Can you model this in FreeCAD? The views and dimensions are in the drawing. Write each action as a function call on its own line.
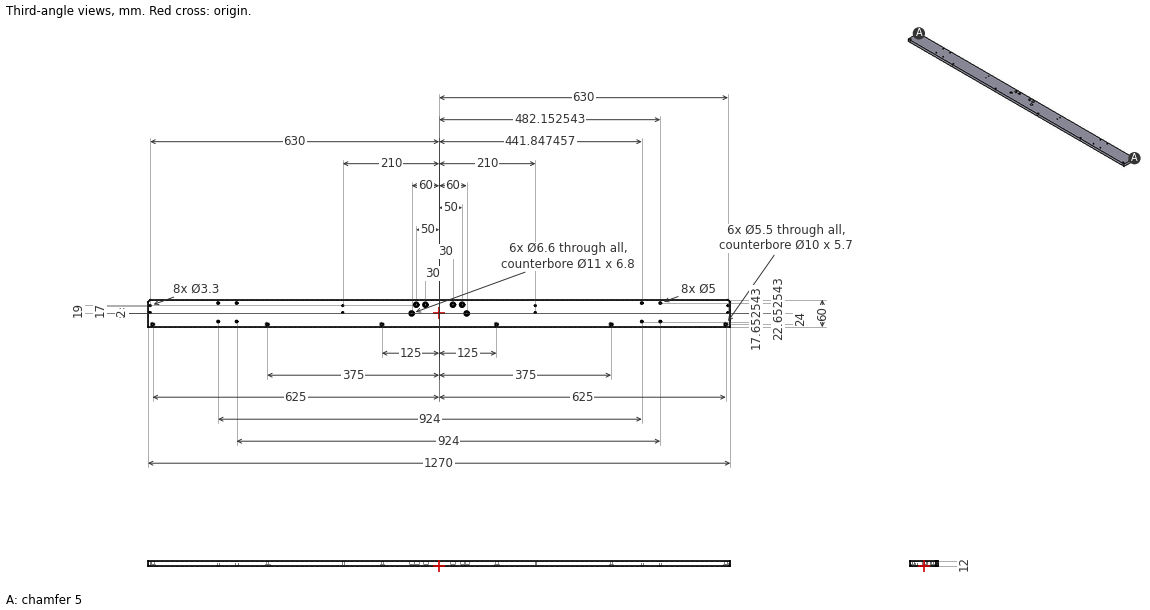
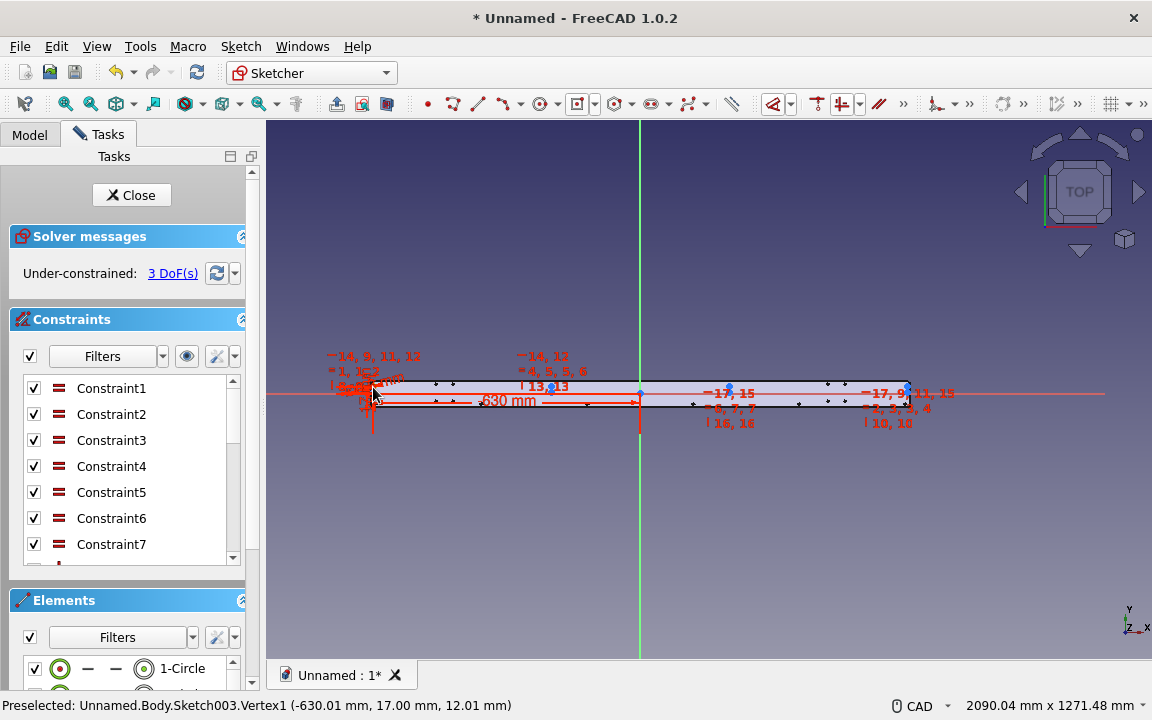
scroll(907, 393, up, 4)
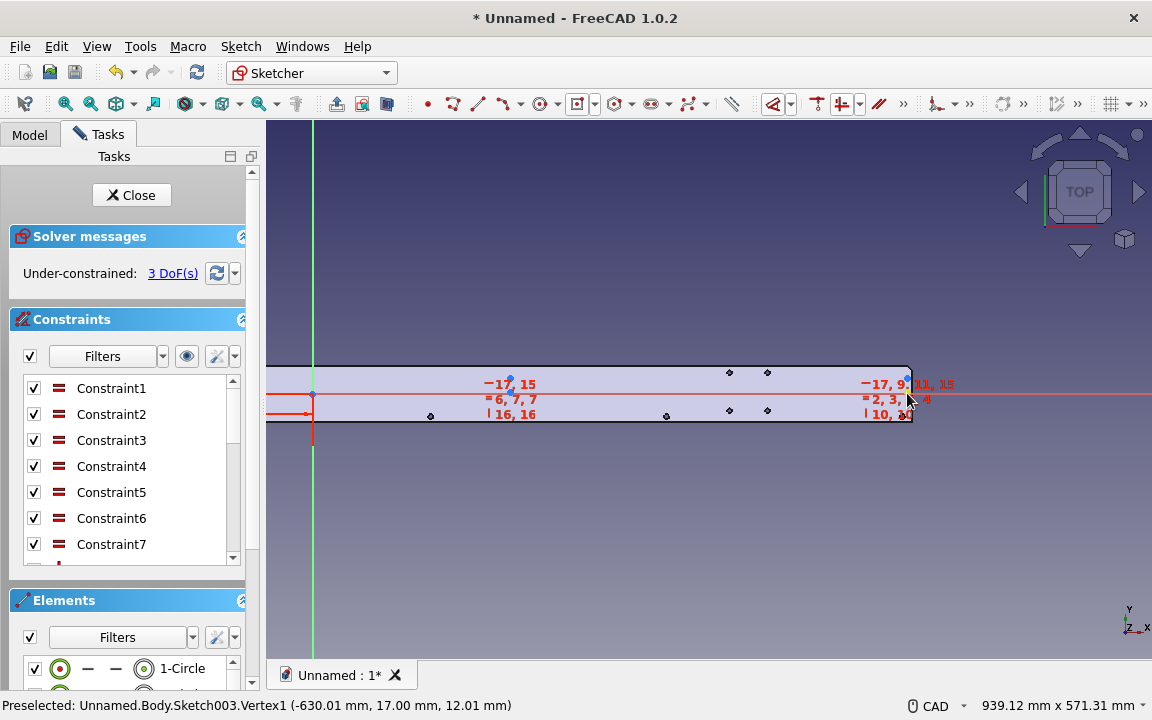
click(907, 392)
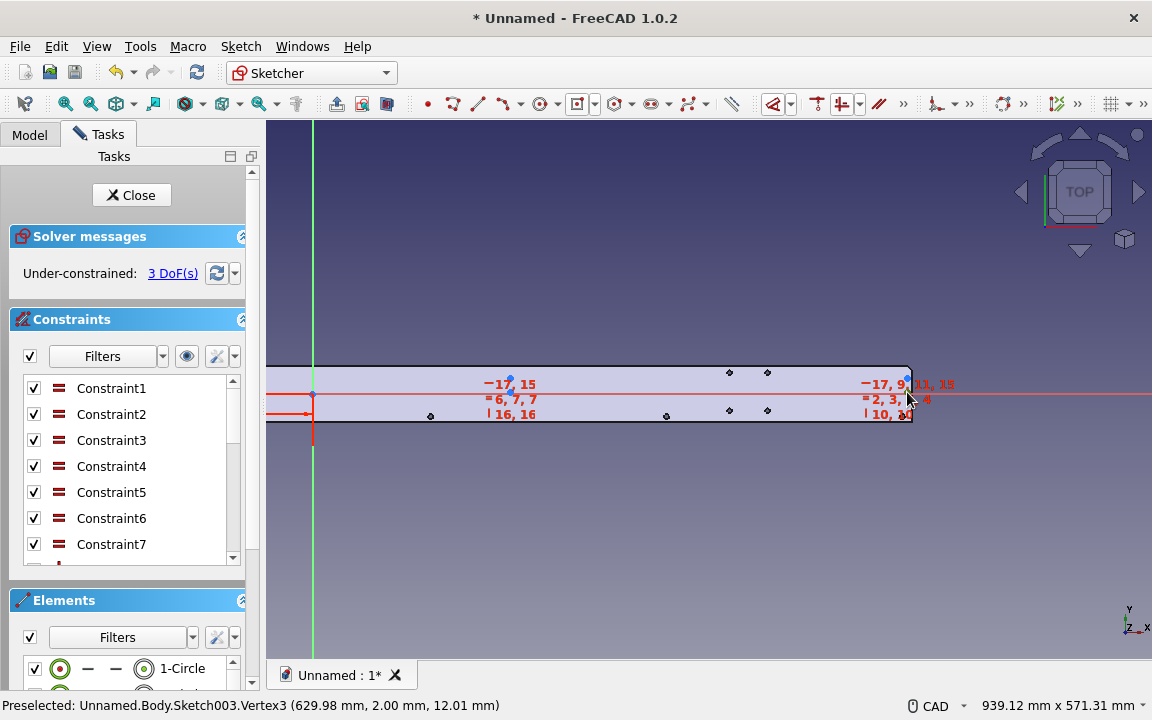
click(790, 104)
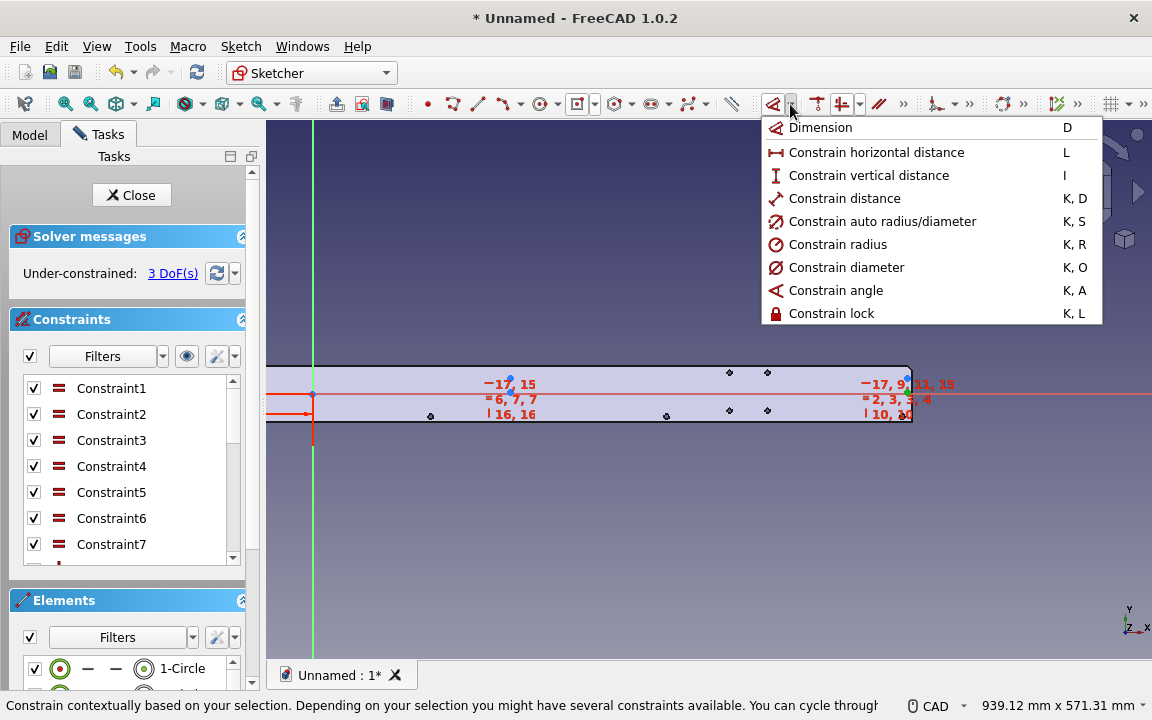
click(932, 152)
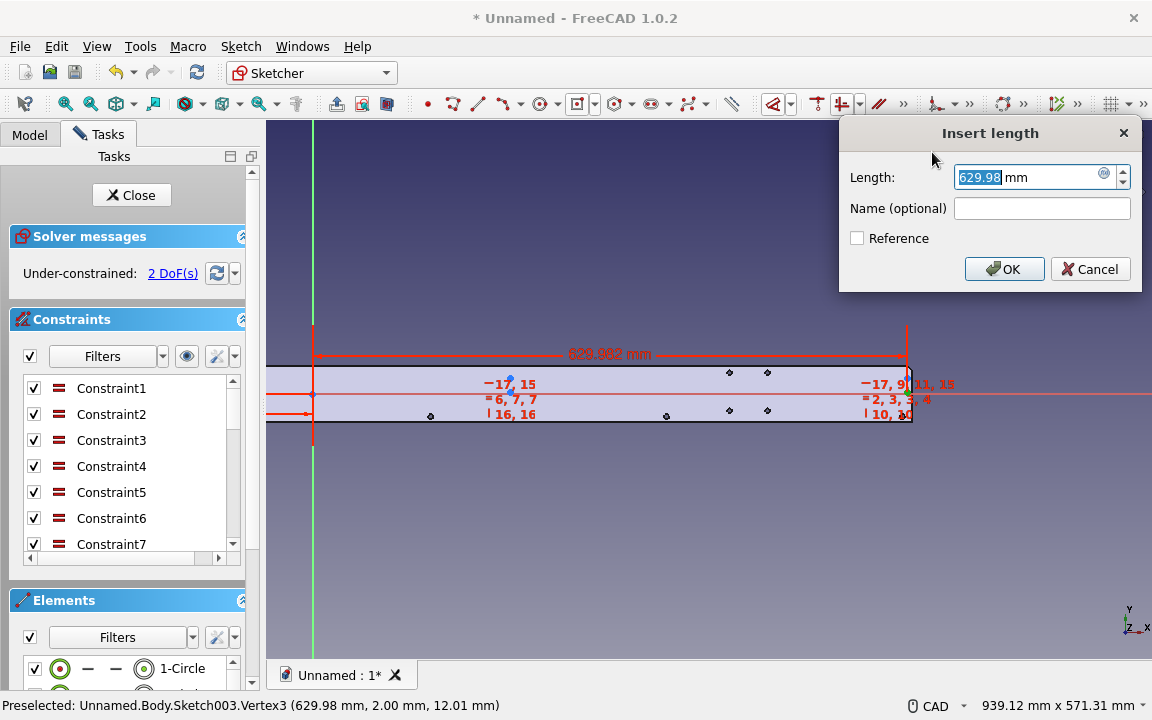
text(630)
key(Return)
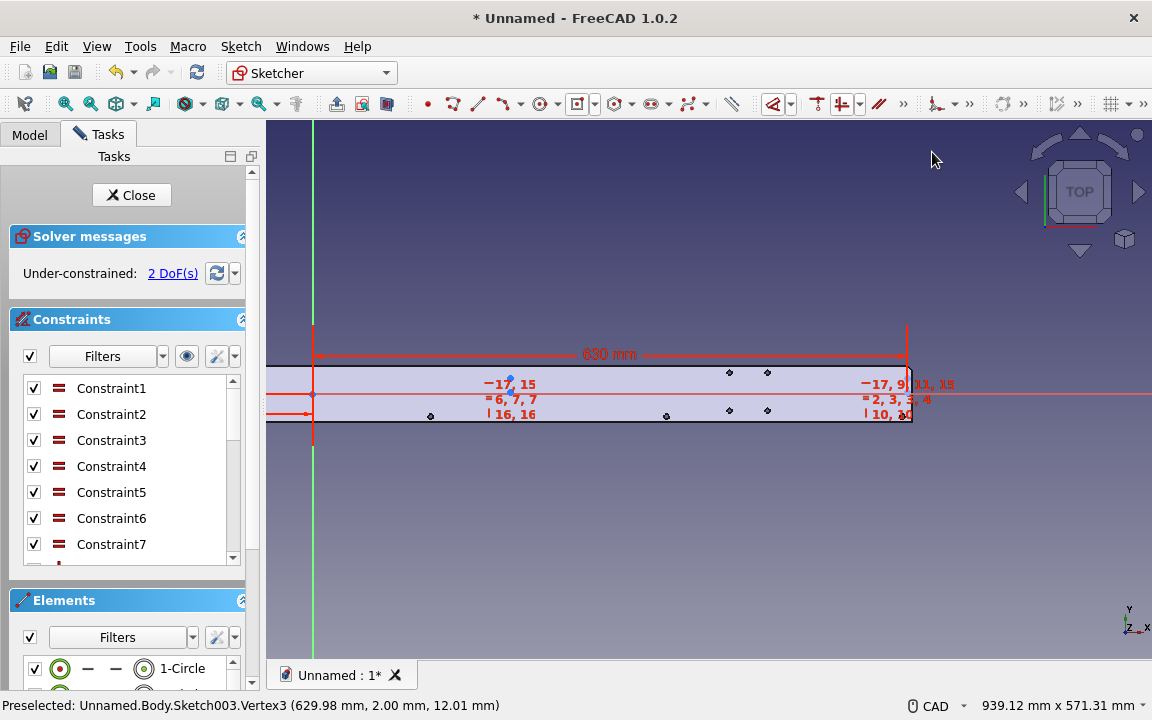
scroll(908, 393, down, 4)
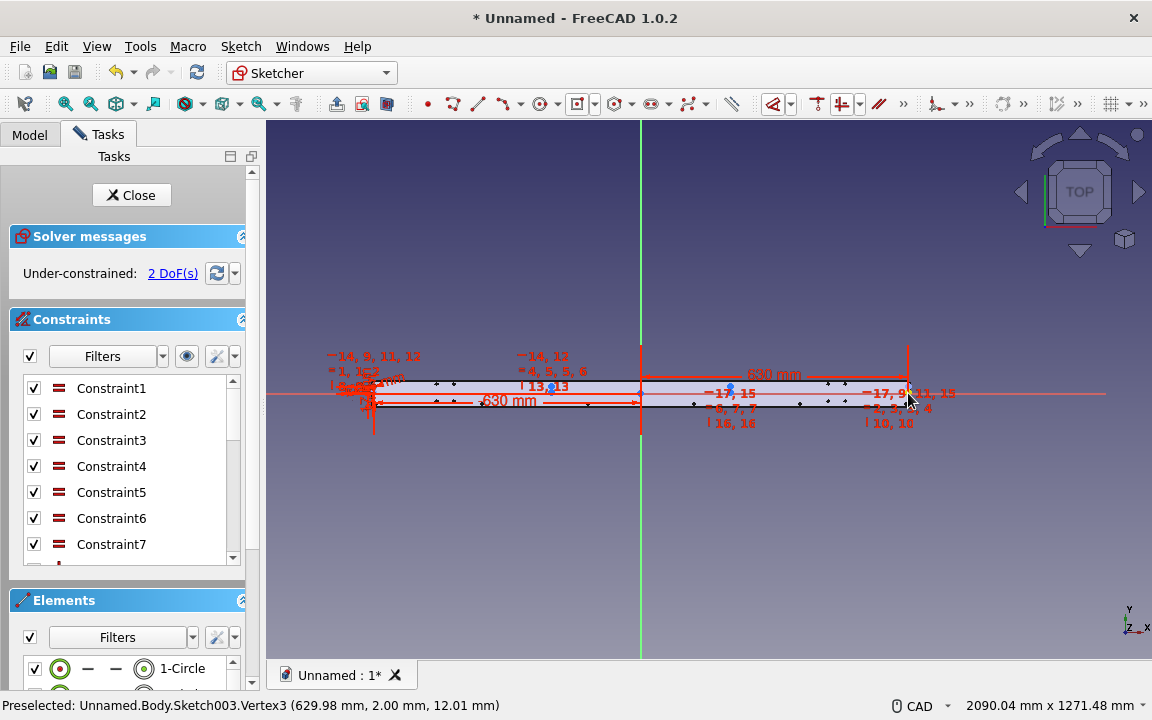
scroll(552, 387, up, 4)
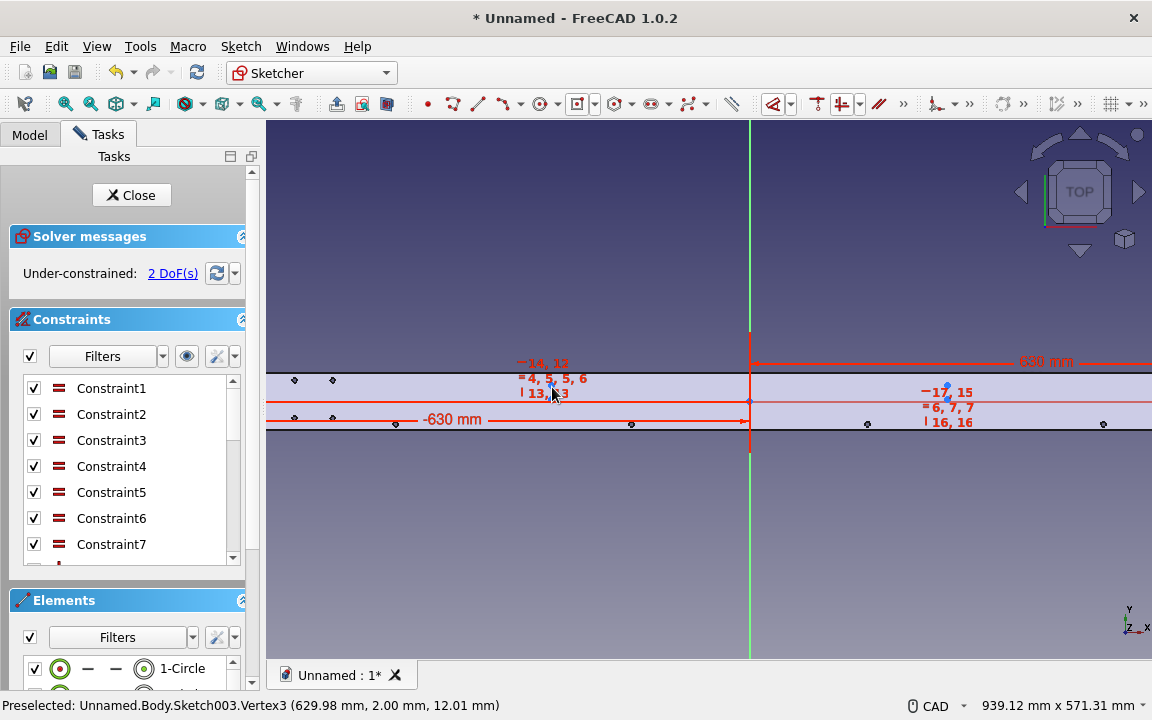
scroll(551, 385, up, 4)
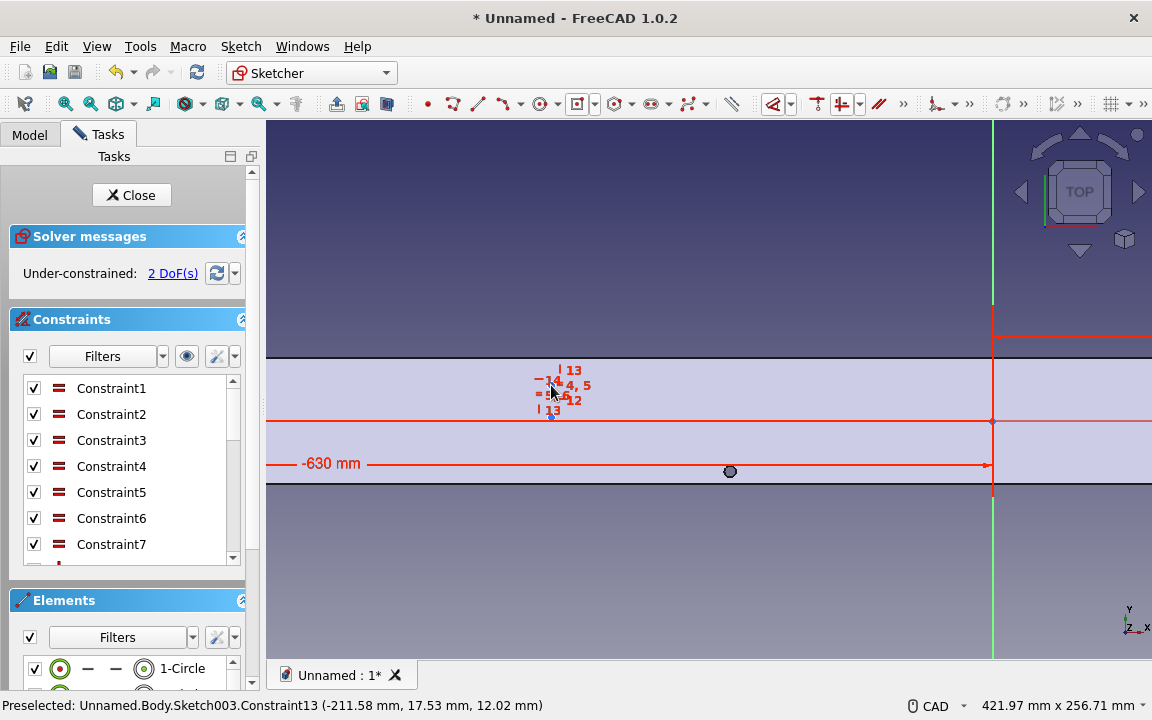
scroll(551, 386, up, 4)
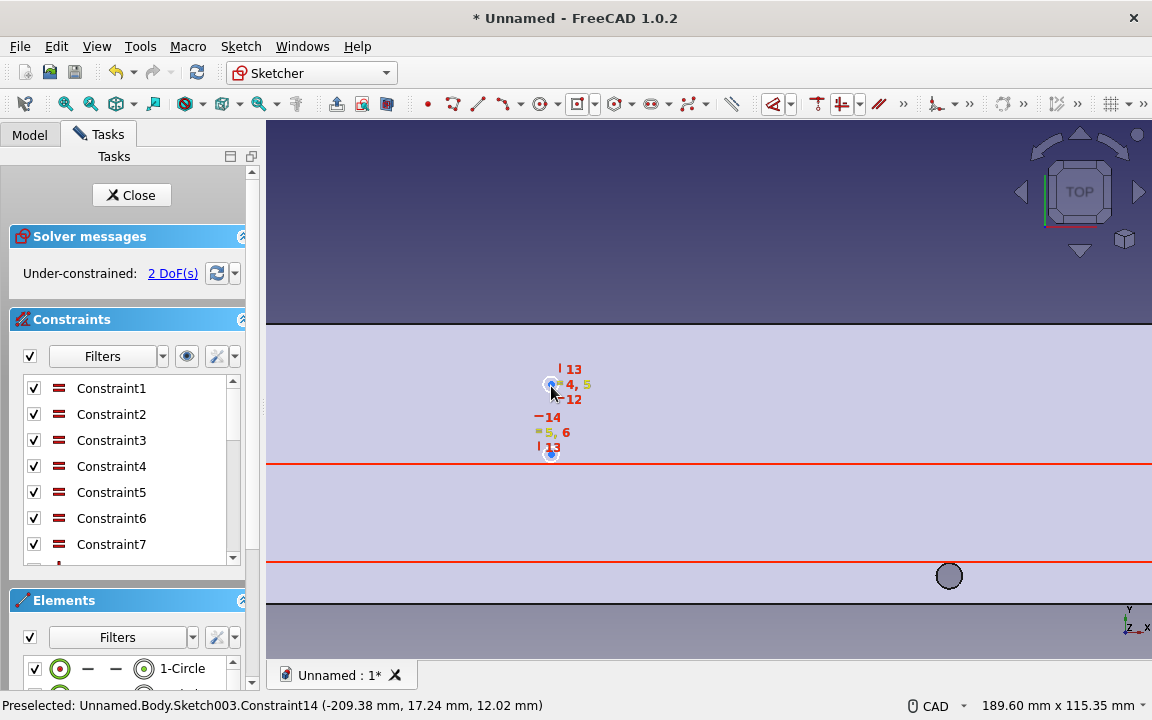
click(551, 384)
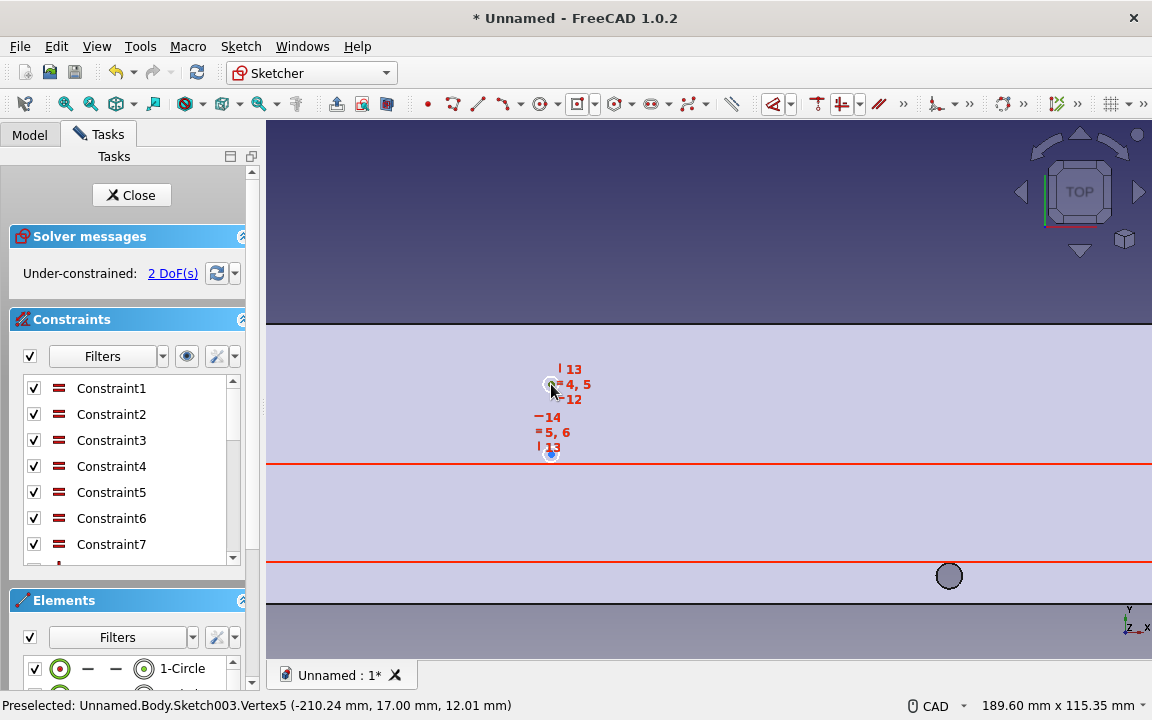
key(l)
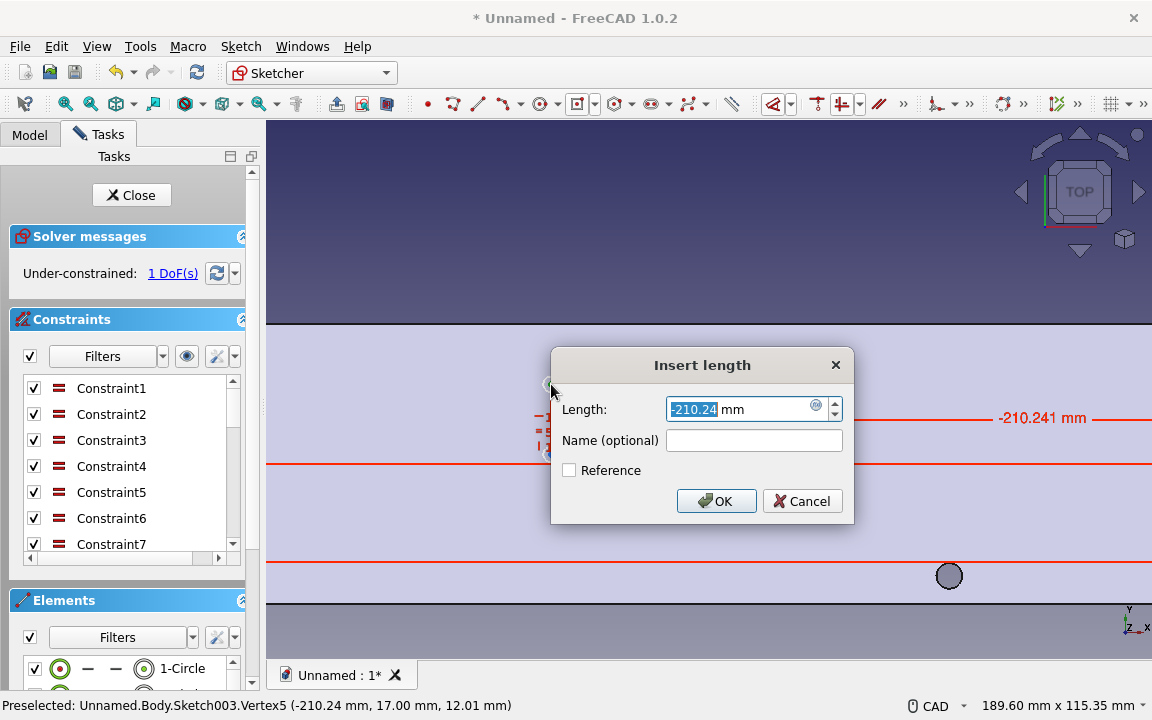
text(-210)
key(Return)